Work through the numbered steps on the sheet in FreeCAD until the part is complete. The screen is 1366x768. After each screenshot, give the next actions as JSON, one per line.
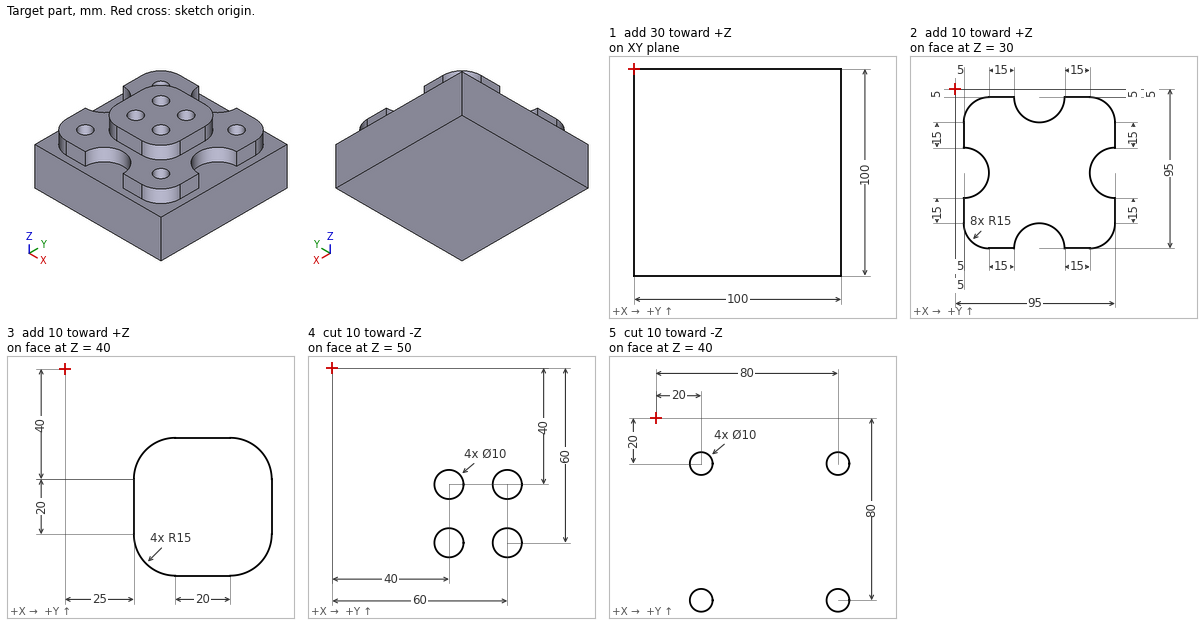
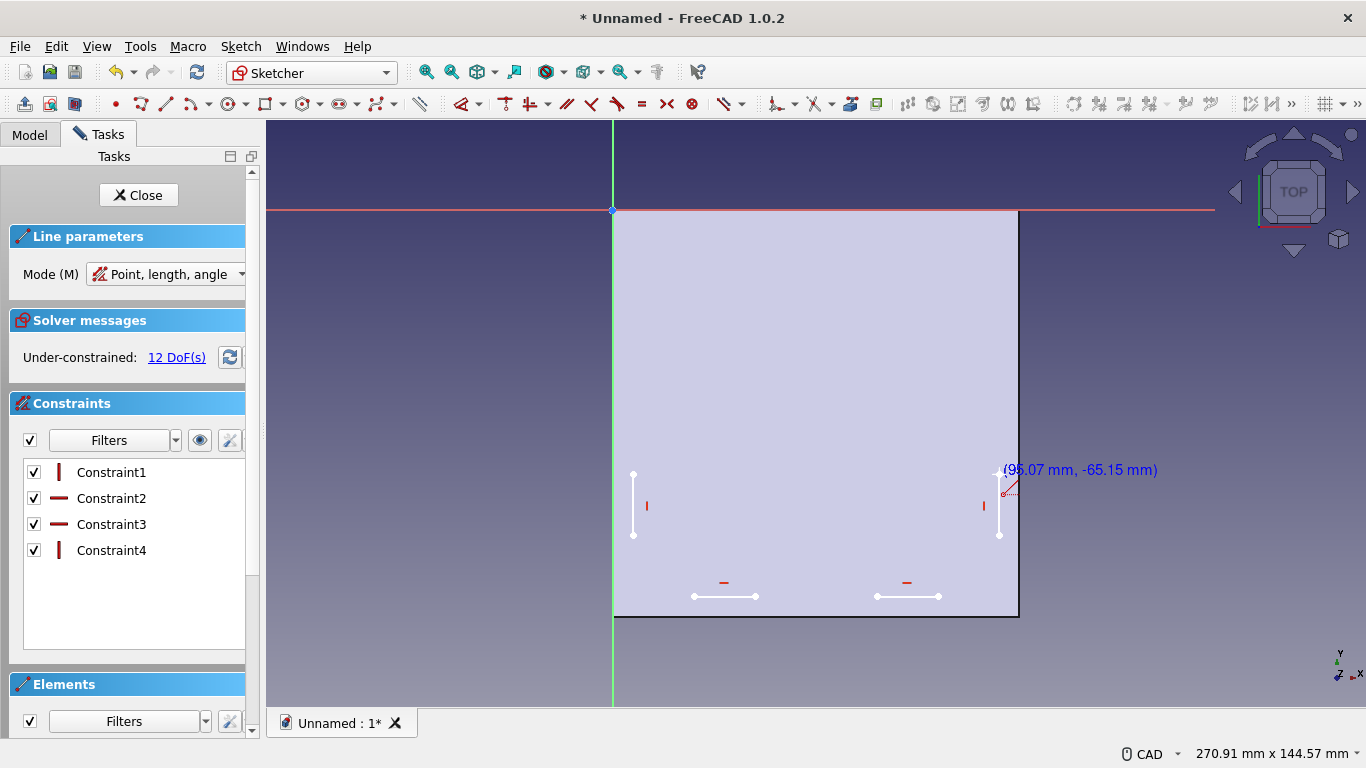
{"action": "left_click", "coordinate": [999, 353]}
{"action": "left_click", "coordinate": [999, 292]}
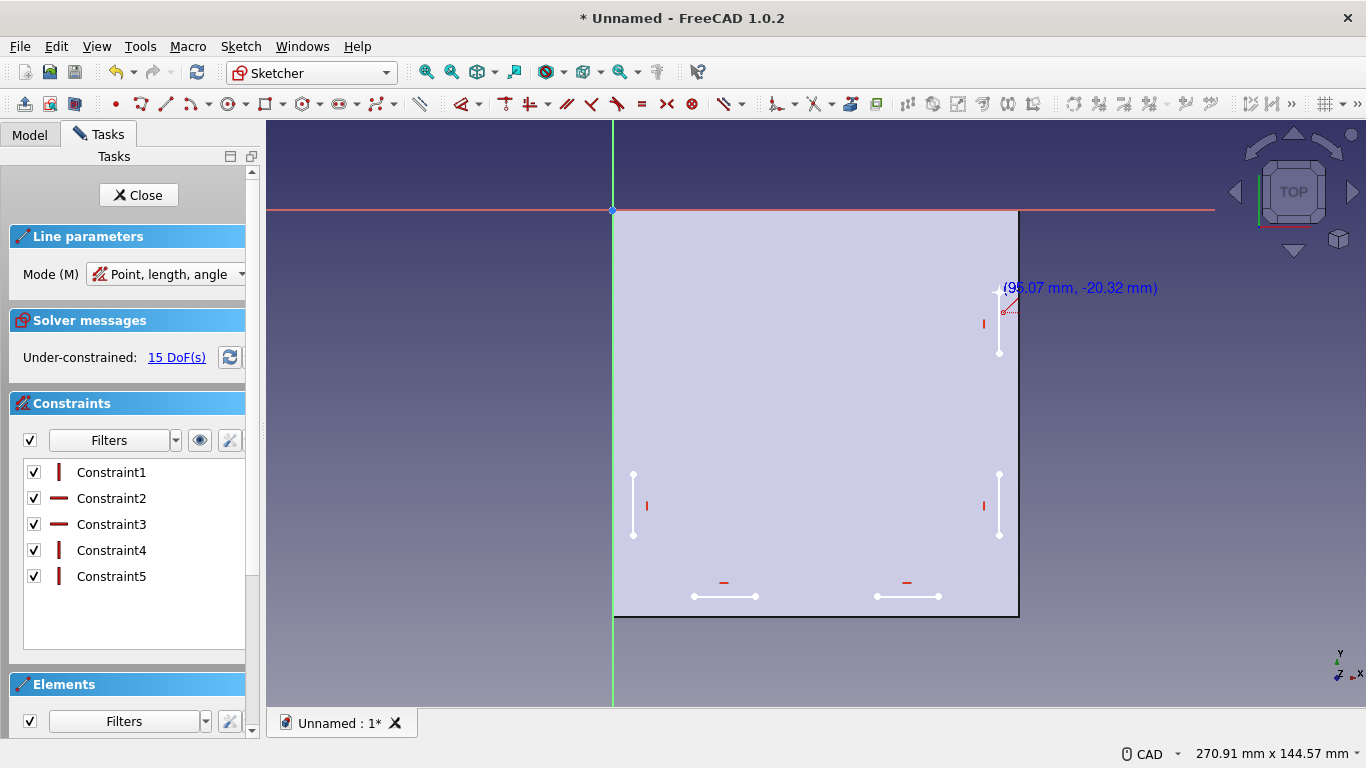
{"action": "left_click", "coordinate": [938, 231]}
{"action": "left_click", "coordinate": [877, 231]}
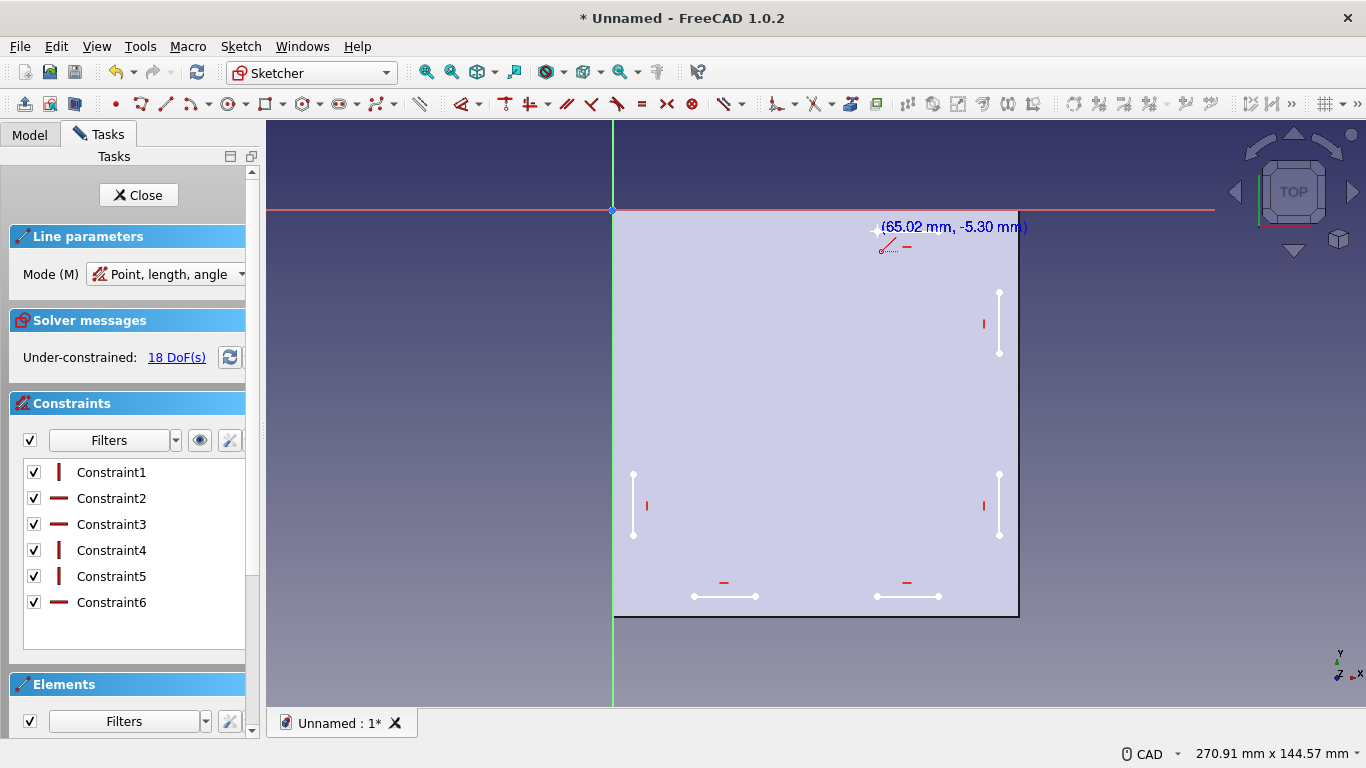
{"action": "left_click", "coordinate": [755, 231]}
{"action": "left_click", "coordinate": [694, 231]}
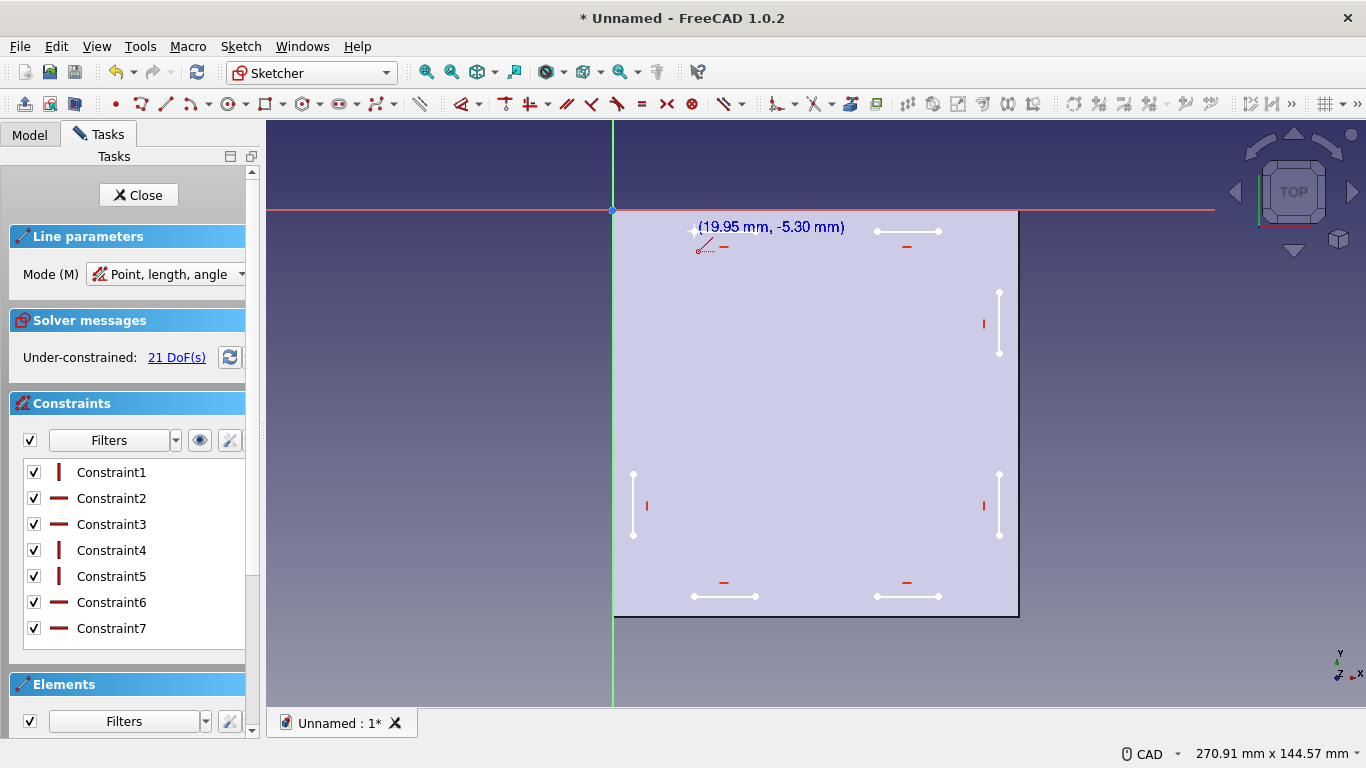
{"action": "left_click", "coordinate": [633, 292]}
{"action": "left_click", "coordinate": [633, 353]}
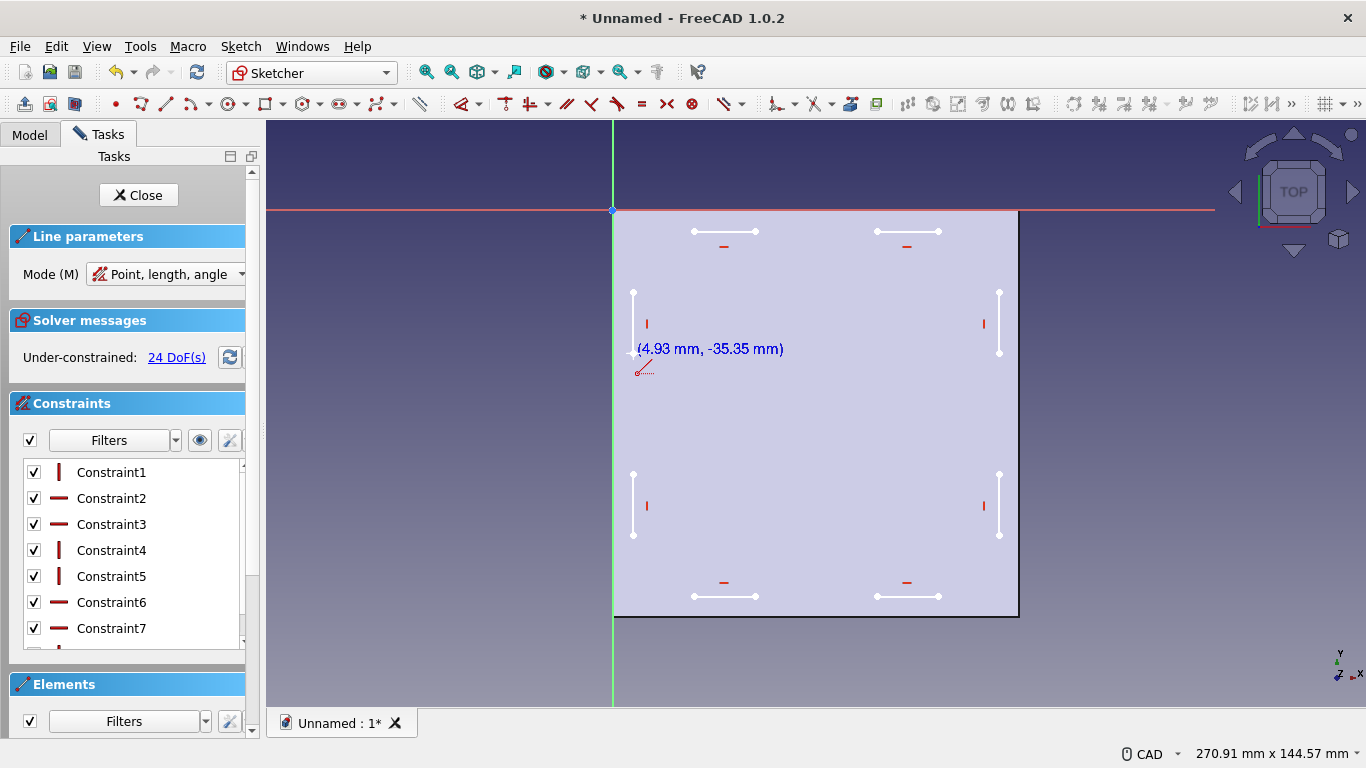
{"action": "key", "text": "g 3 a"}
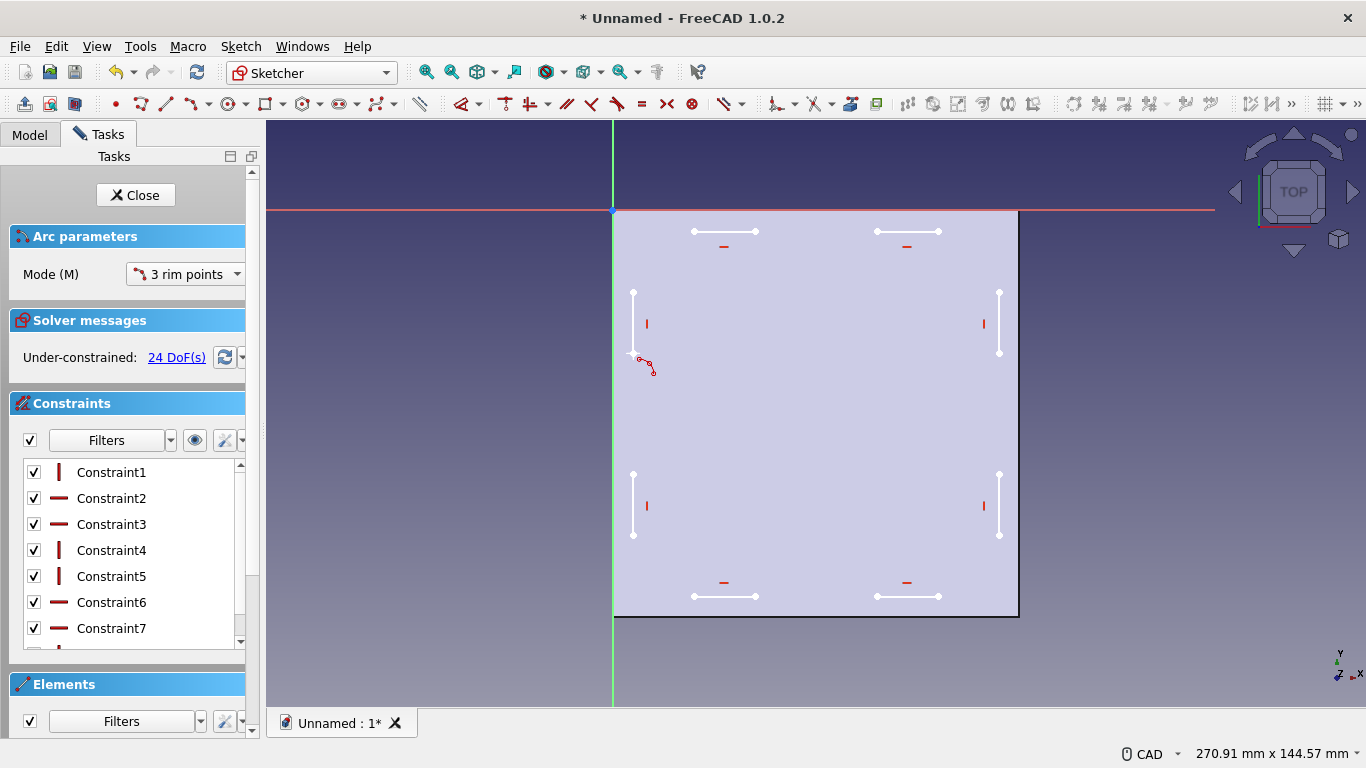
{"action": "left_click", "coordinate": [633, 536]}
{"action": "left_click", "coordinate": [694, 597]}
{"action": "left_click", "coordinate": [651, 578]}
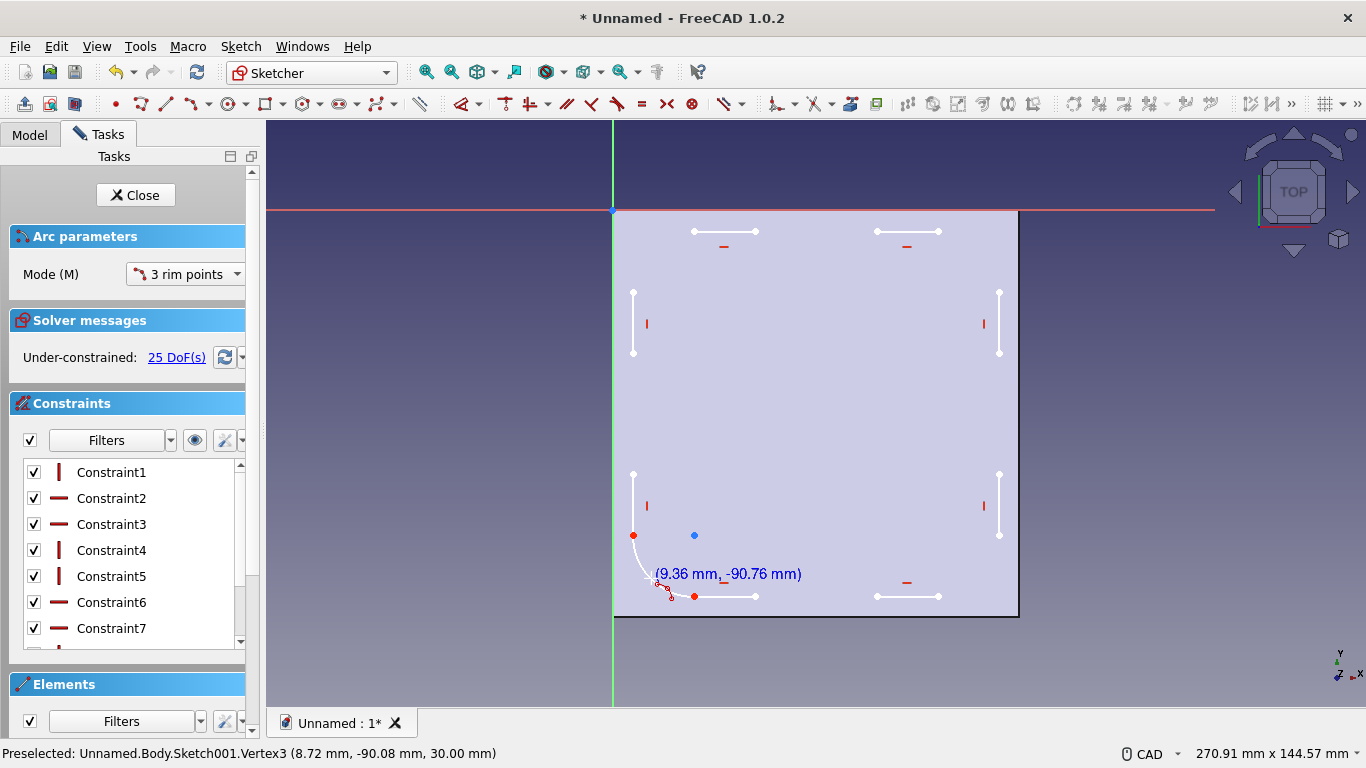
{"action": "left_click", "coordinate": [755, 597]}
{"action": "left_click", "coordinate": [877, 597]}
{"action": "left_click", "coordinate": [816, 535]}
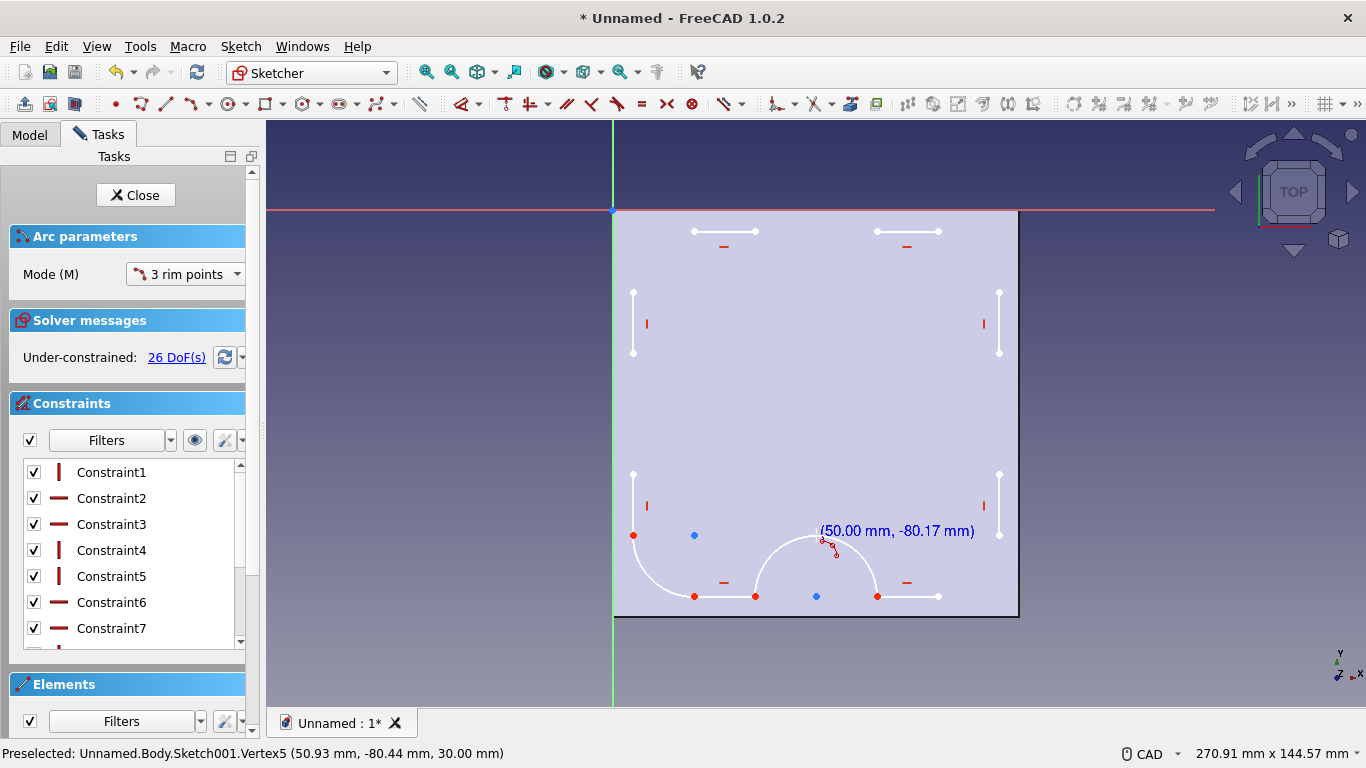
{"action": "left_click", "coordinate": [938, 597]}
{"action": "left_click", "coordinate": [999, 536]}
{"action": "left_click", "coordinate": [981, 578]}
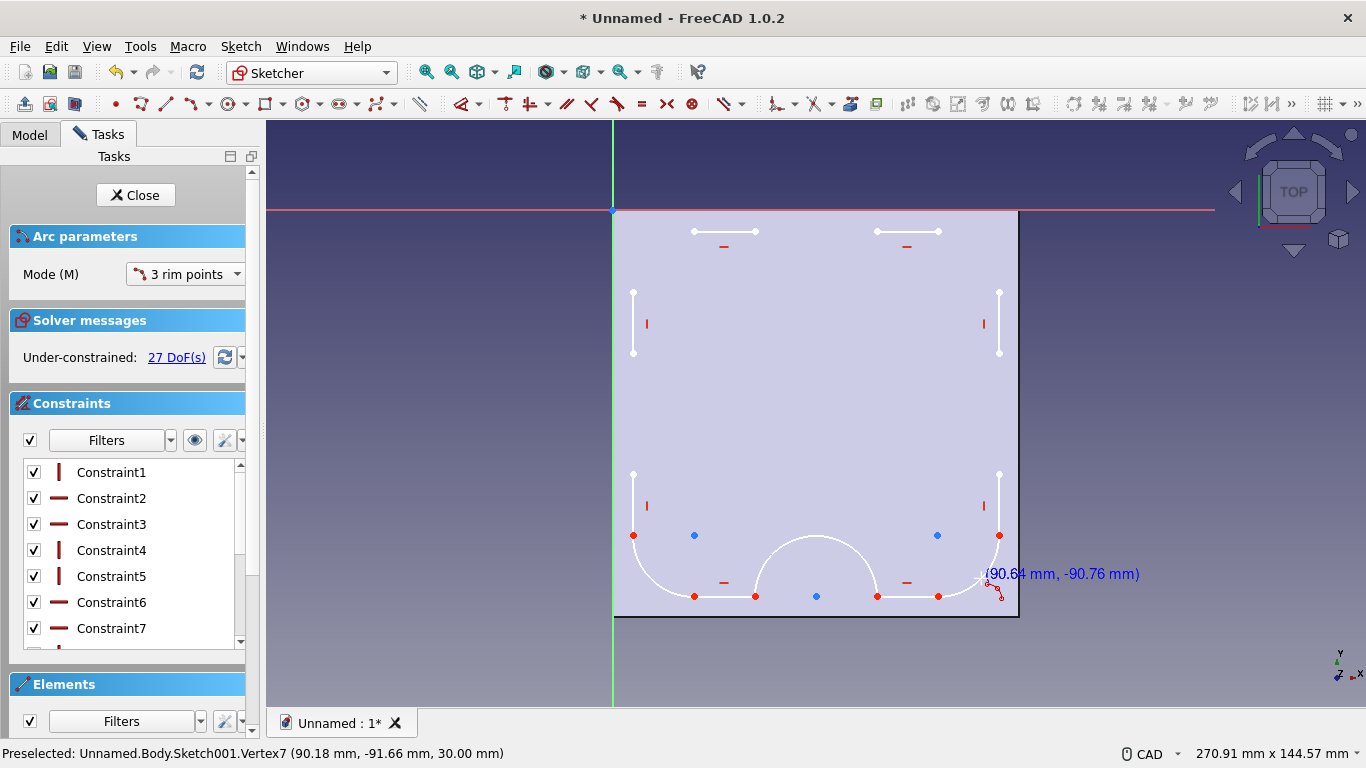
{"action": "left_click", "coordinate": [999, 475]}
{"action": "left_click", "coordinate": [999, 354]}
{"action": "left_click", "coordinate": [938, 413]}